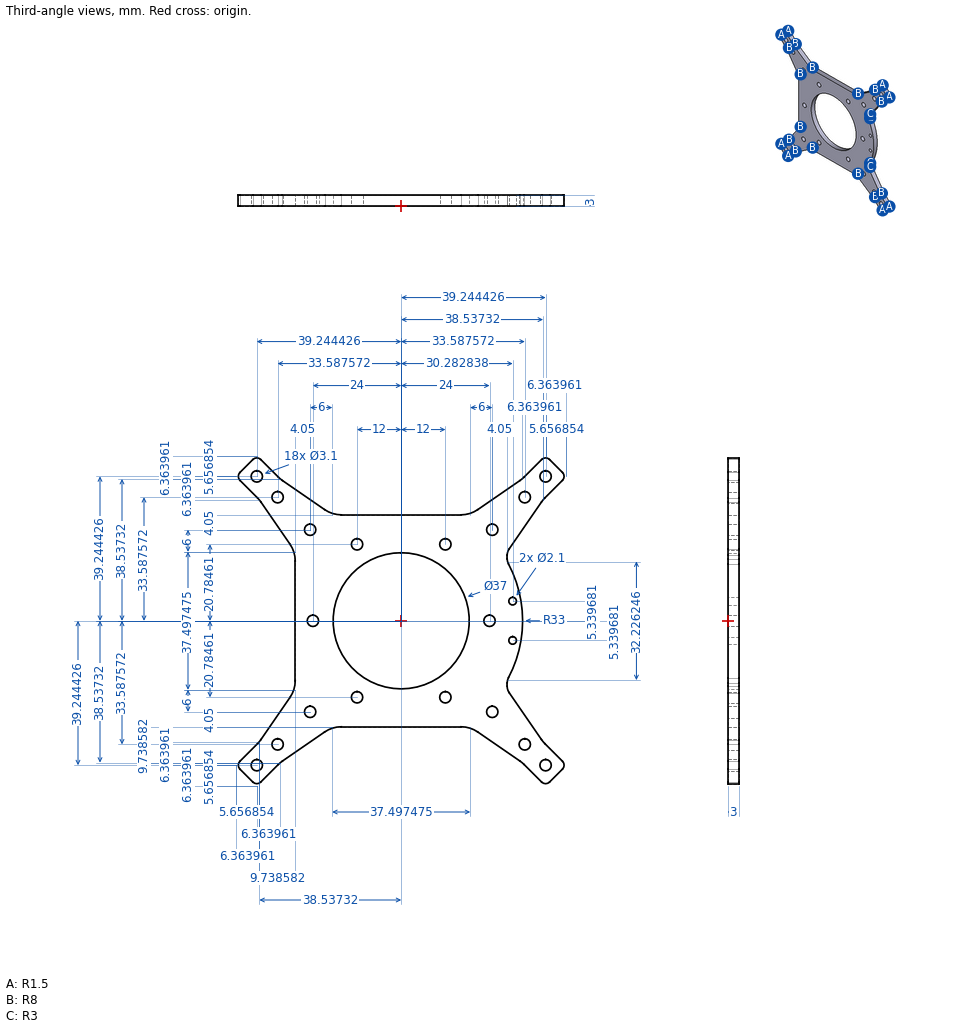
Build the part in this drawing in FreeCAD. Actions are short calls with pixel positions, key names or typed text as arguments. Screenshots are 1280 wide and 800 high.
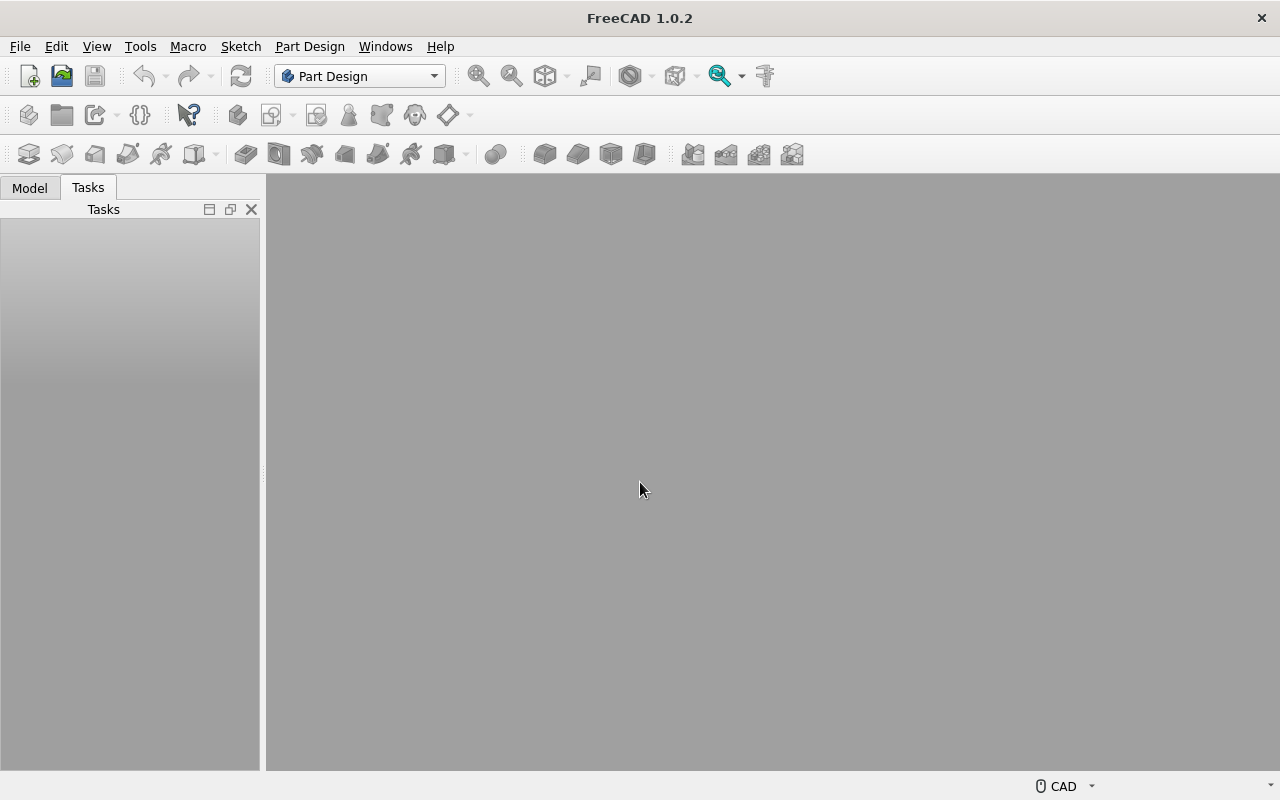
click(29, 76)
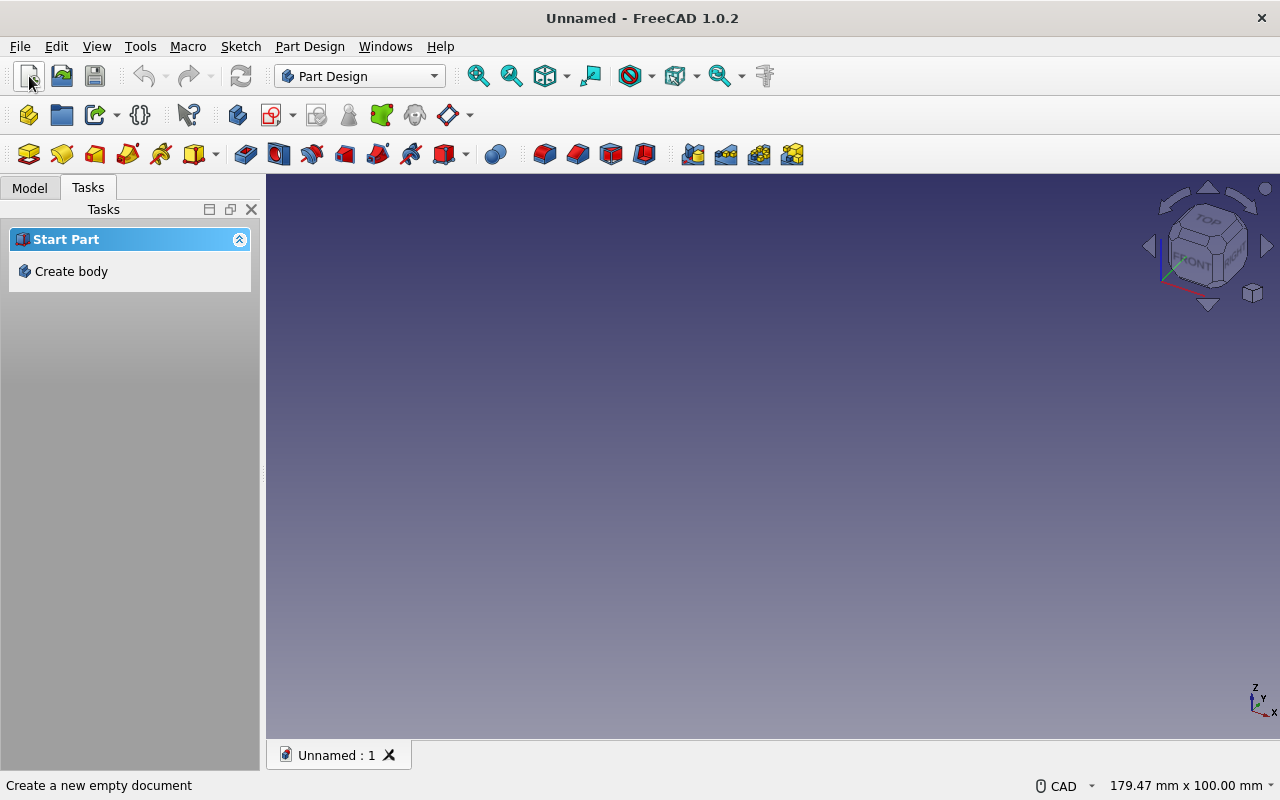
click(270, 116)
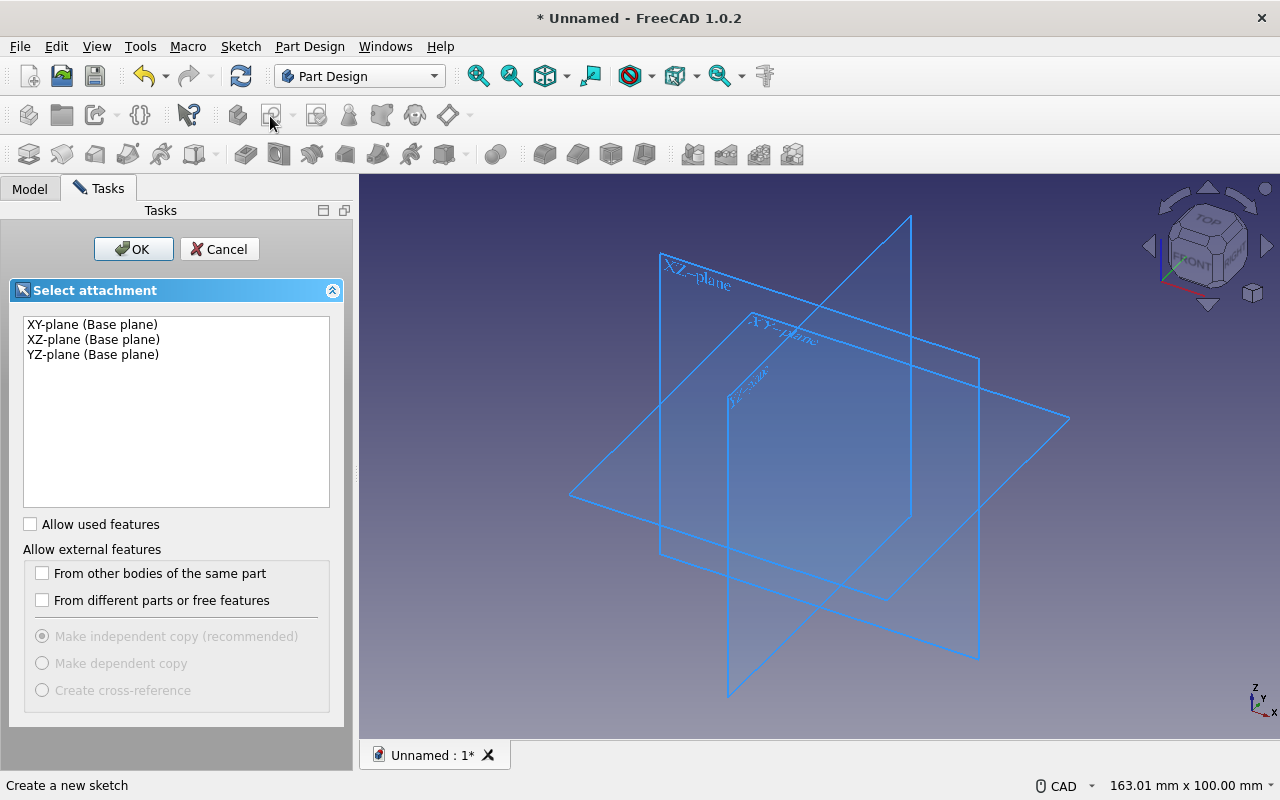
click(84, 340)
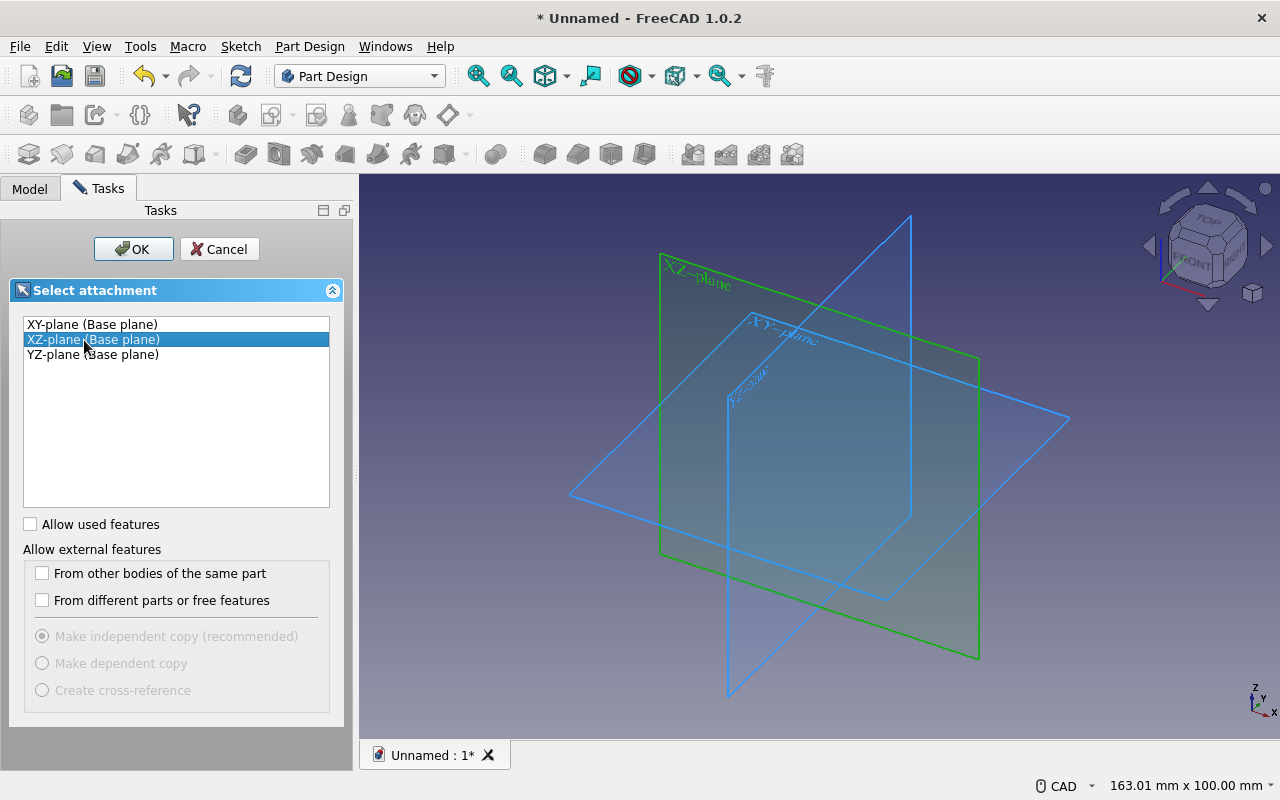
click(134, 249)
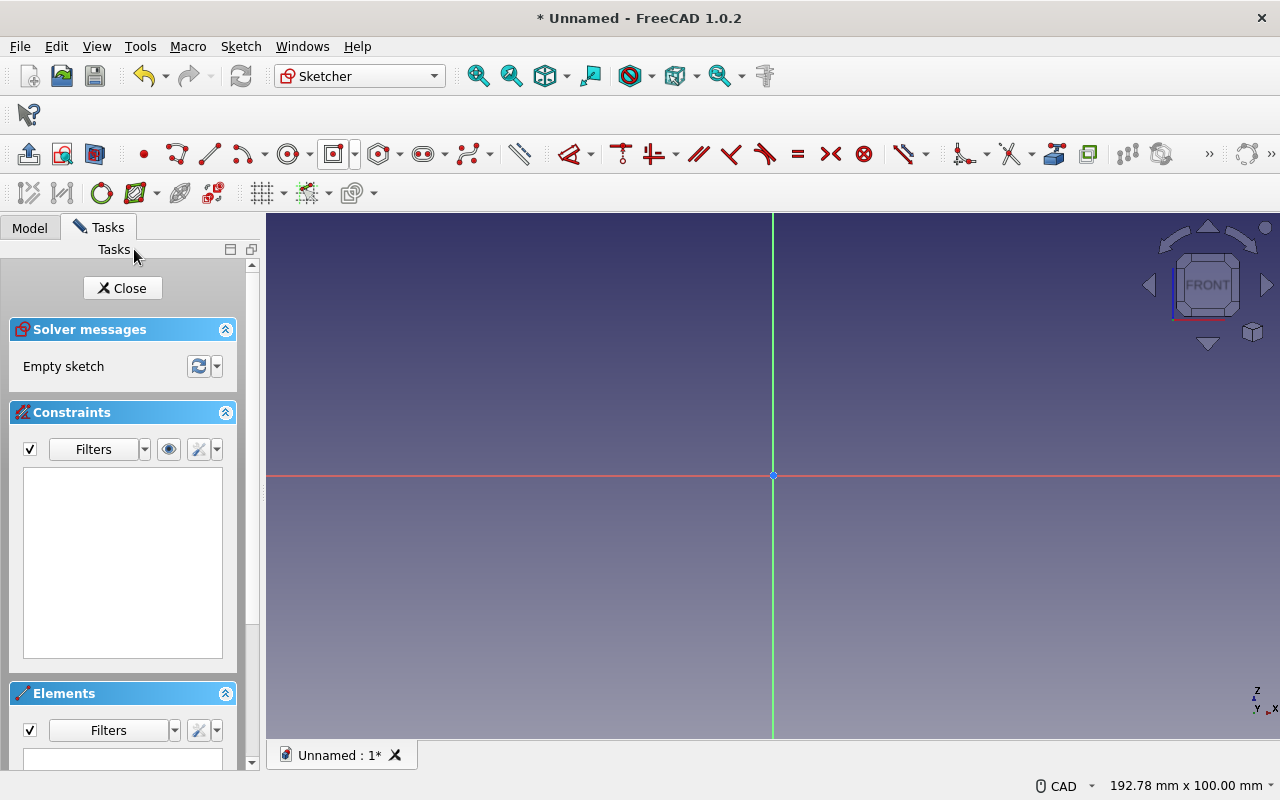
scroll(565, 476, down, 2)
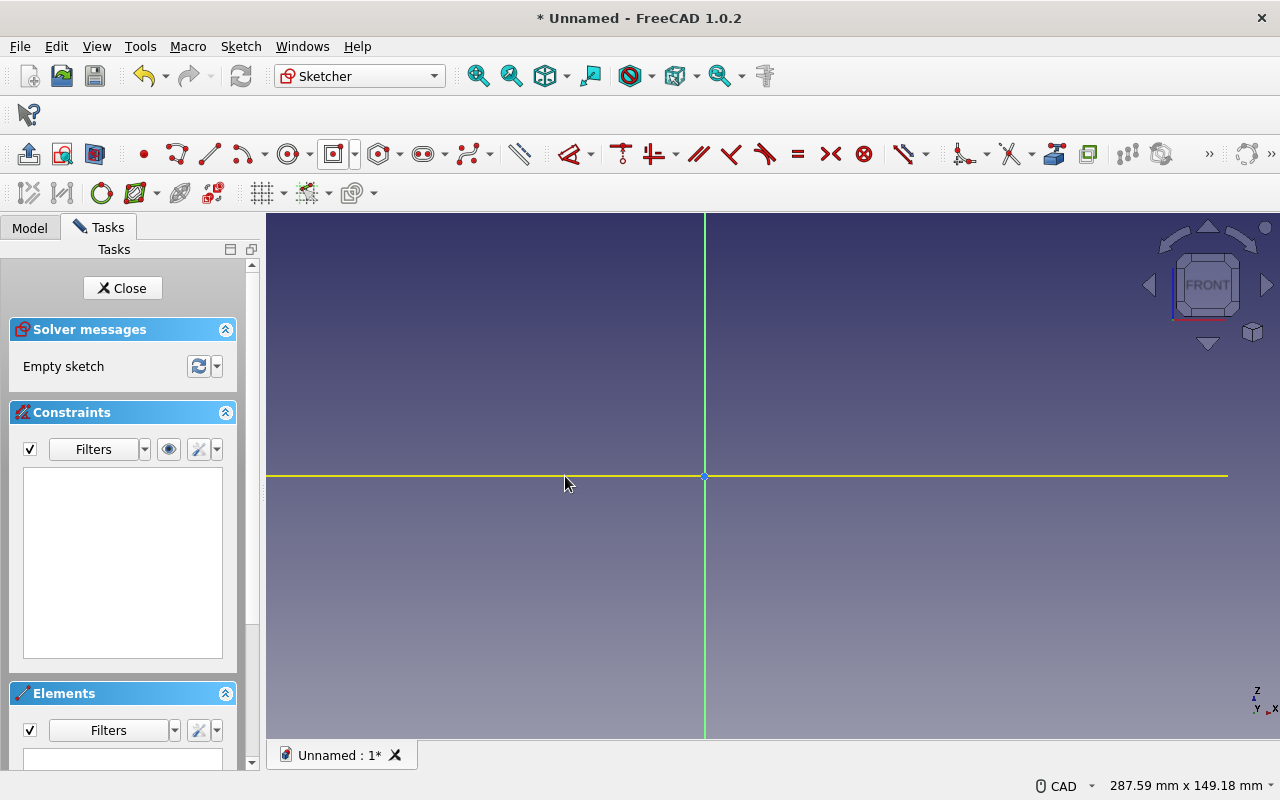
click(177, 154)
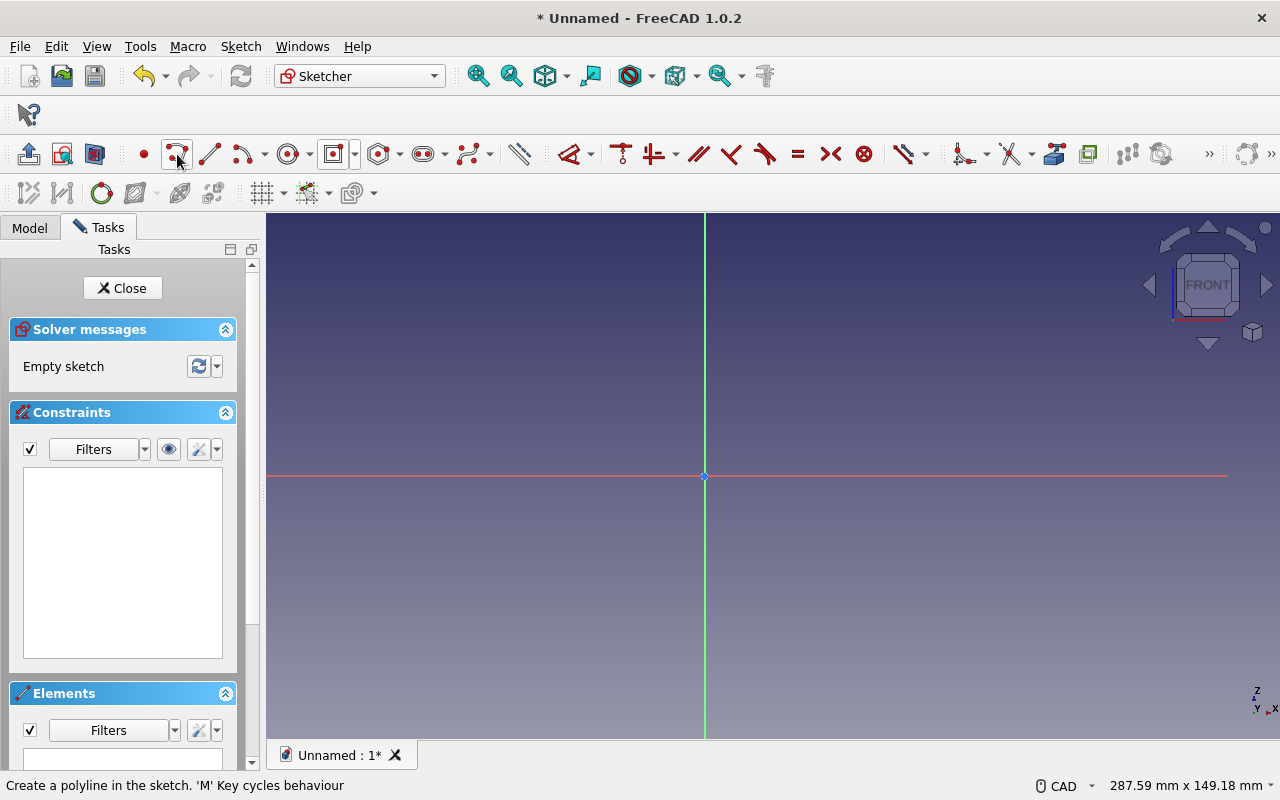
click(771, 578)
click(638, 578)
click(589, 612)
click(566, 634)
click(546, 615)
click(569, 592)
click(603, 542)
click(603, 410)
click(569, 360)
click(546, 338)
click(566, 318)
click(589, 340)
click(638, 375)
click(771, 375)
click(820, 340)
click(843, 318)
click(863, 338)
click(840, 360)
click(806, 410)
click(806, 542)
click(840, 592)
click(863, 615)
click(843, 634)
click(820, 612)
click(771, 579)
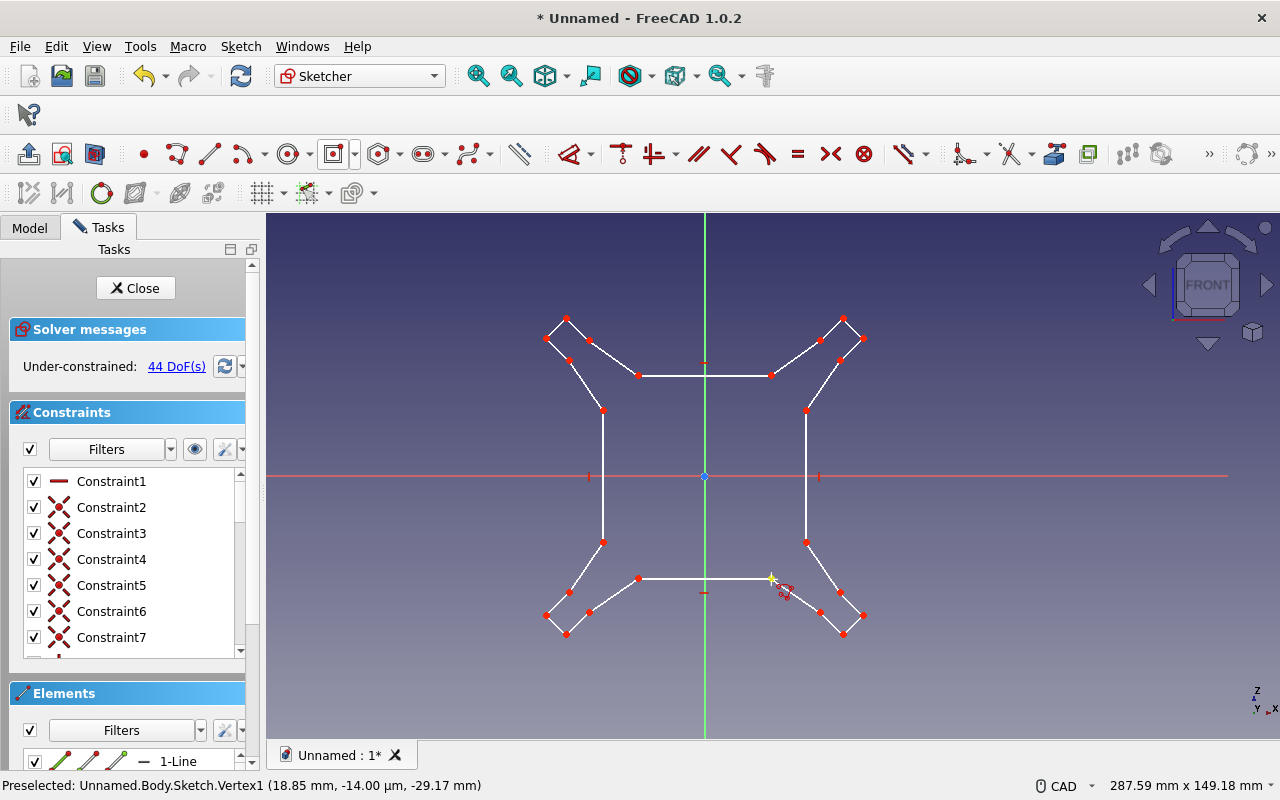
click(288, 154)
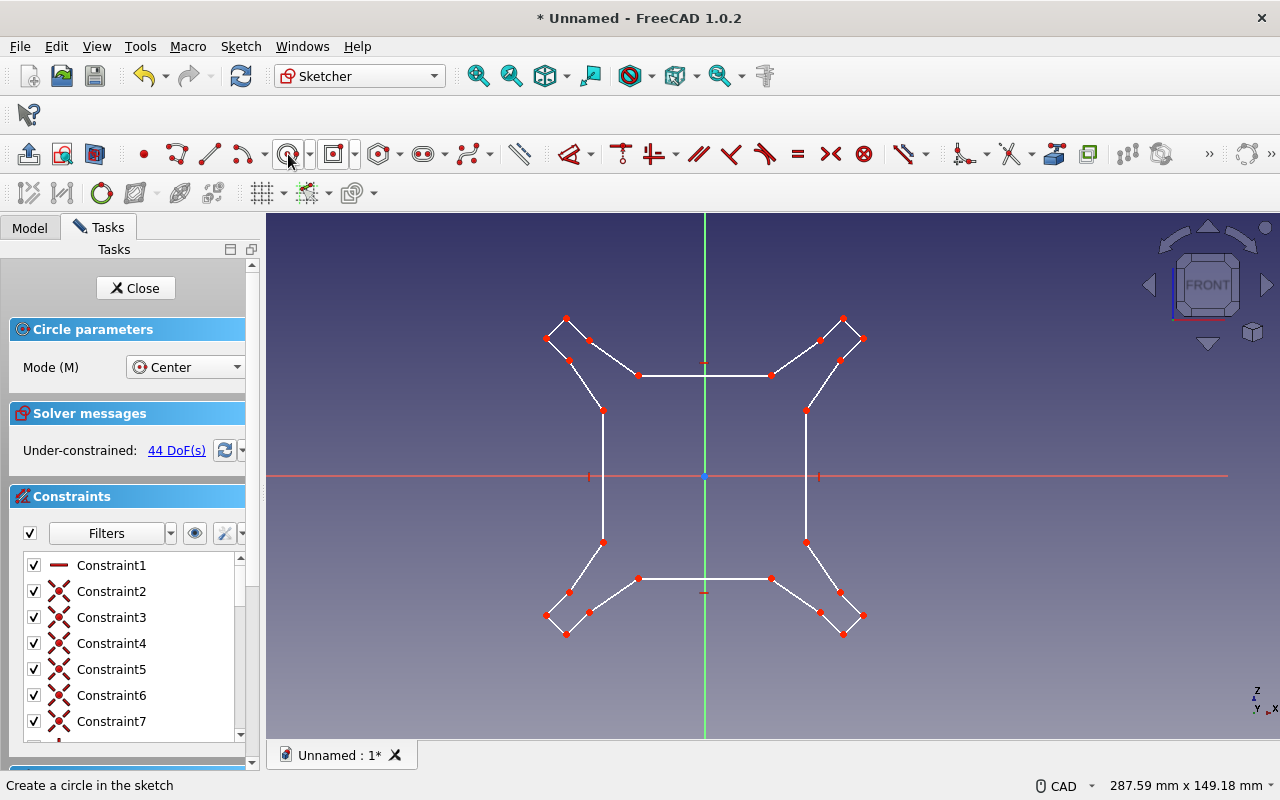
scroll(566, 338, up, 8)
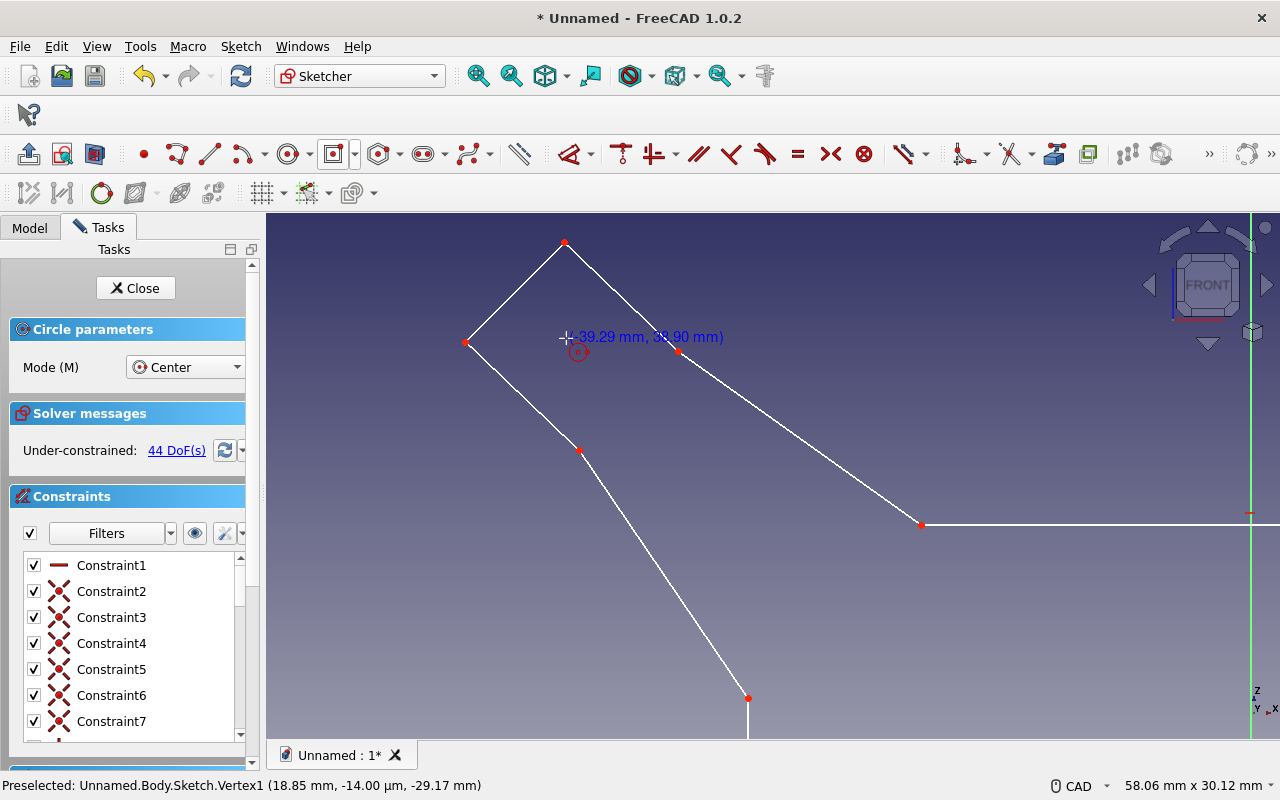
scroll(566, 338, down, 8)